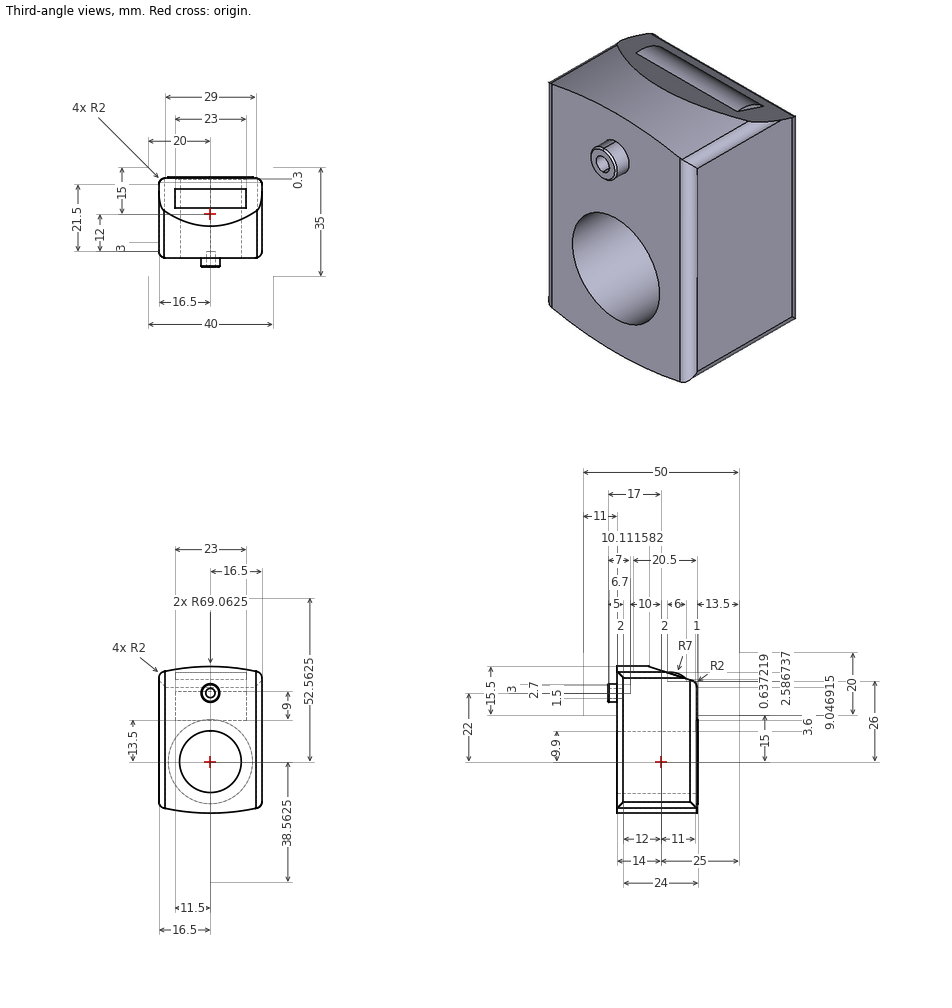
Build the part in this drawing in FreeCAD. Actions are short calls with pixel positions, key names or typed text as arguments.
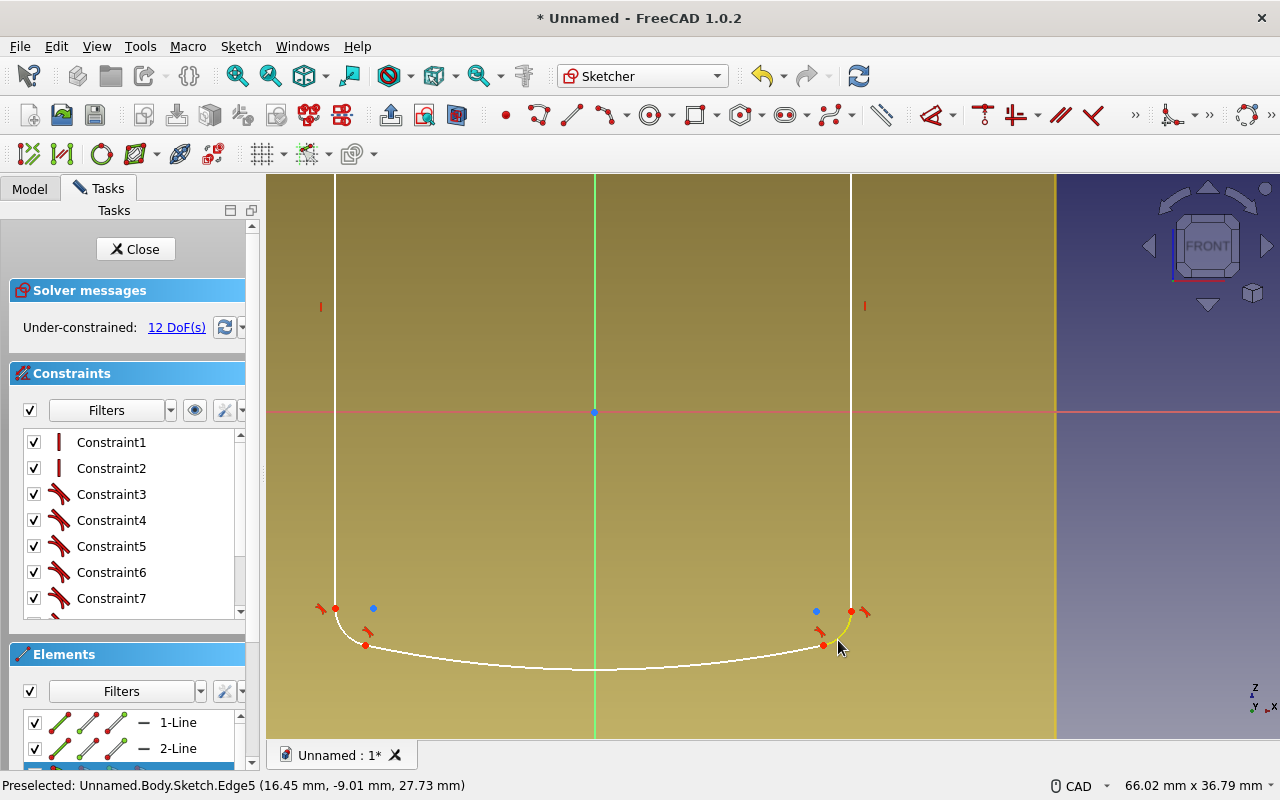
click(837, 640)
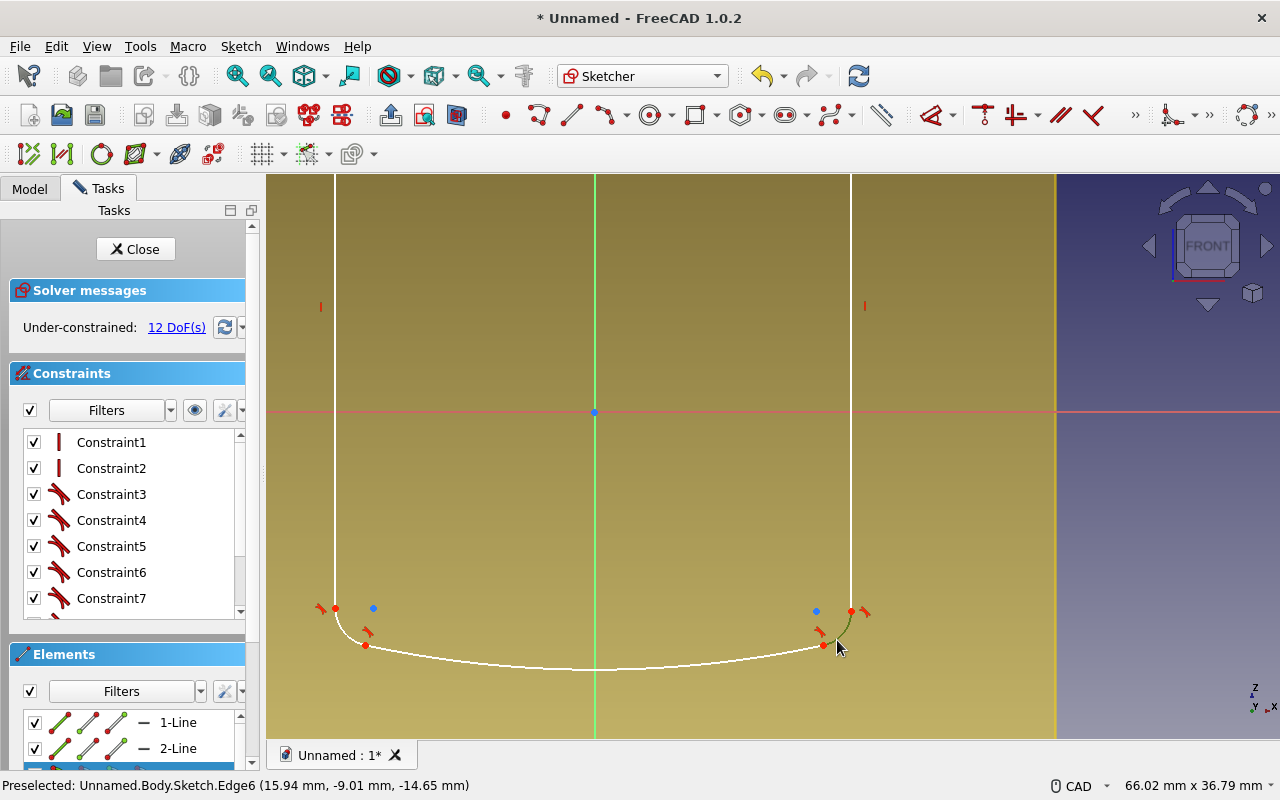
click(339, 623)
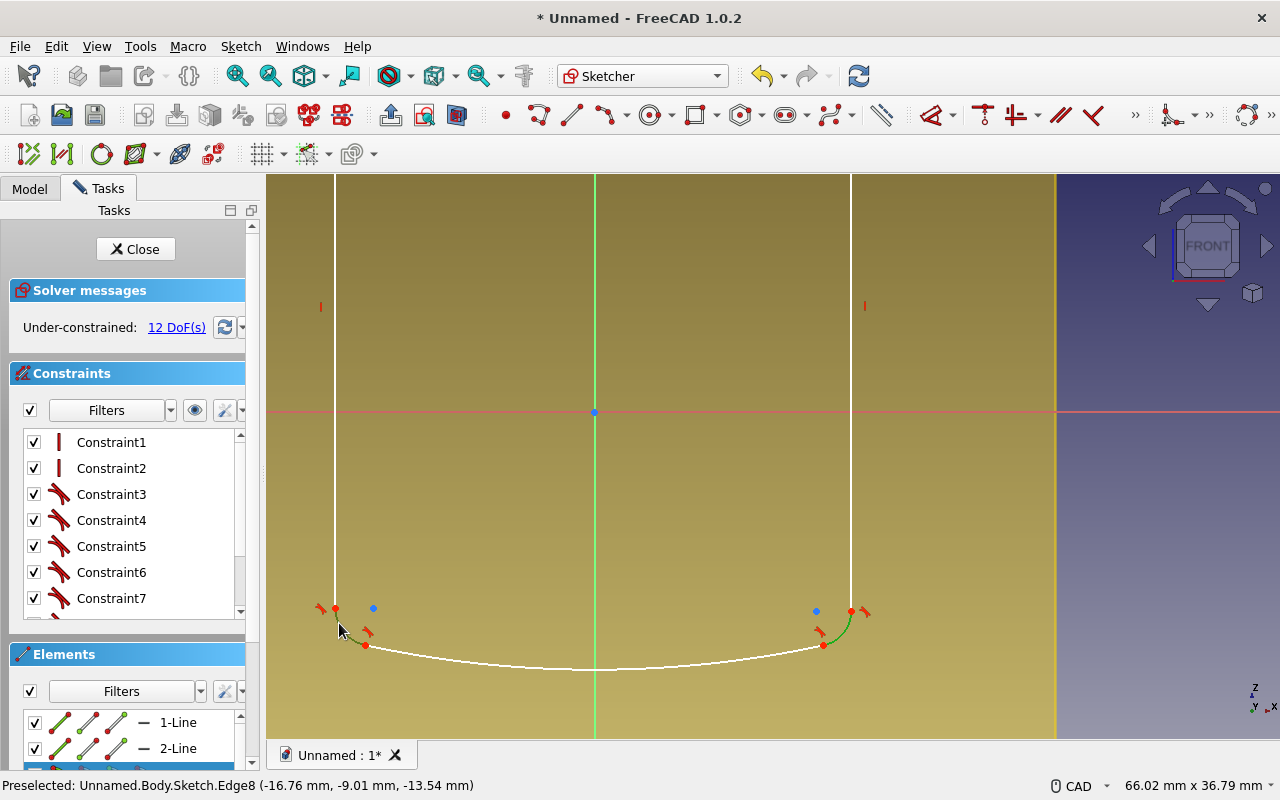
key(e)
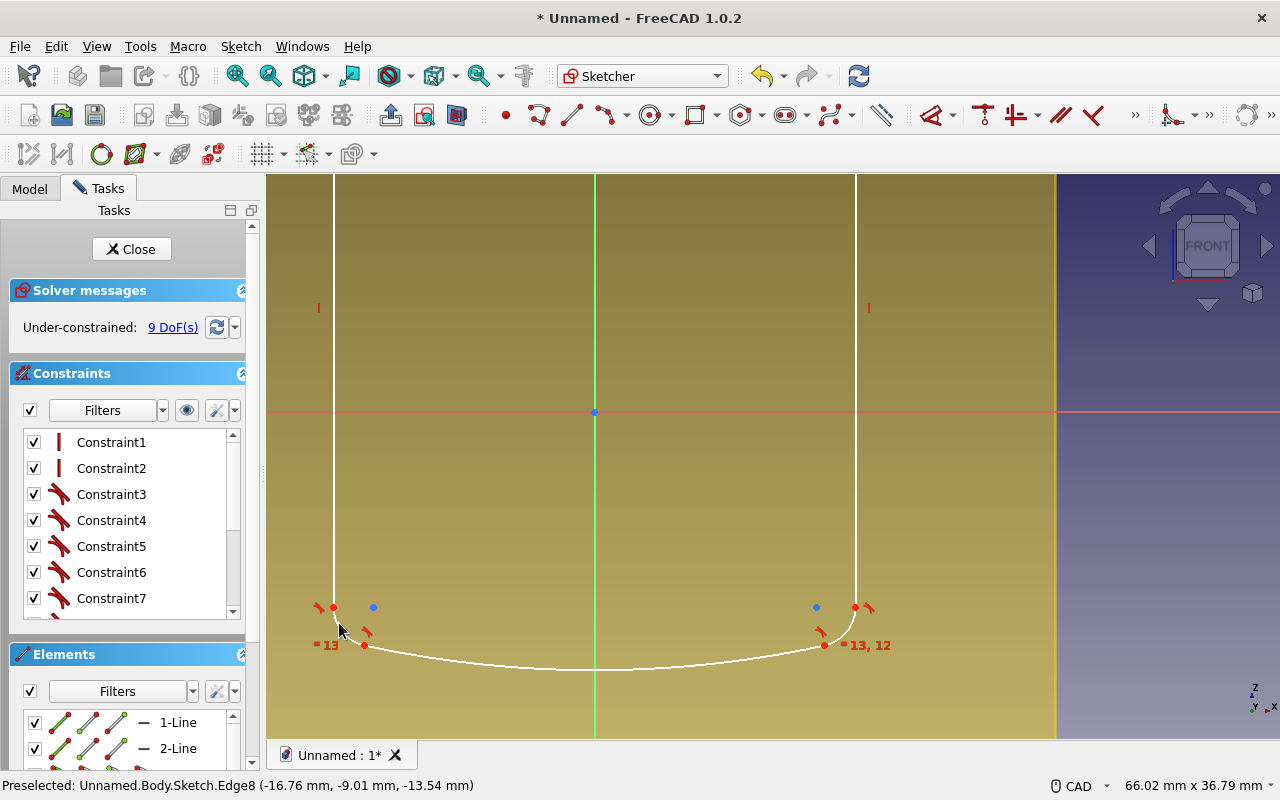
scroll(838, 641, down, 3)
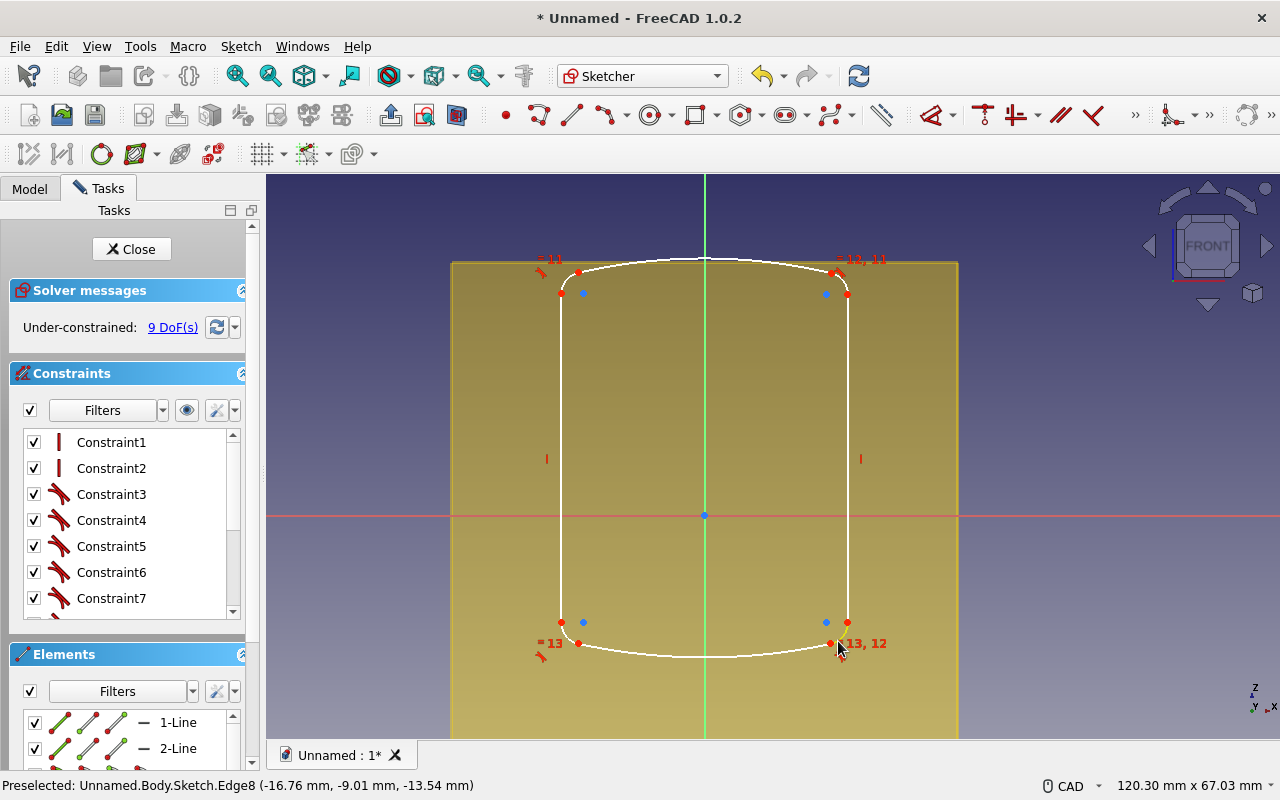
click(756, 261)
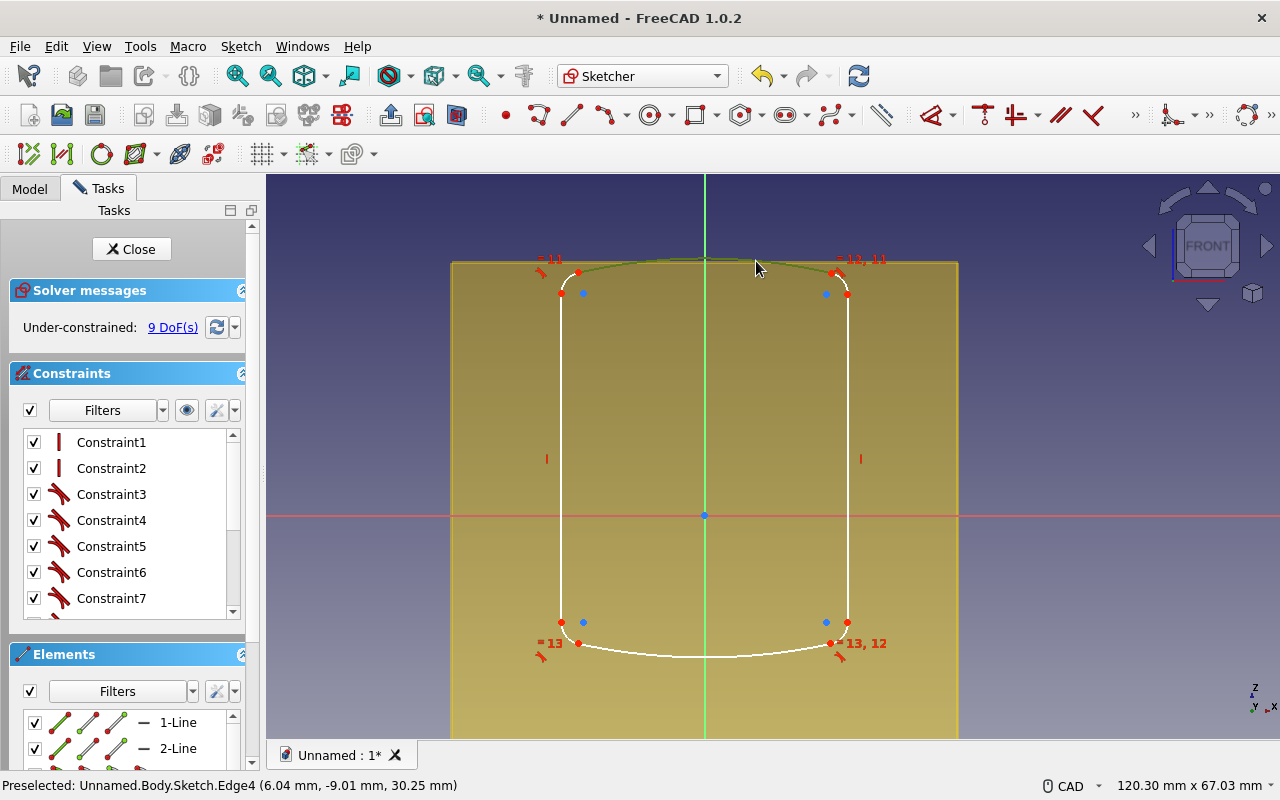
click(654, 655)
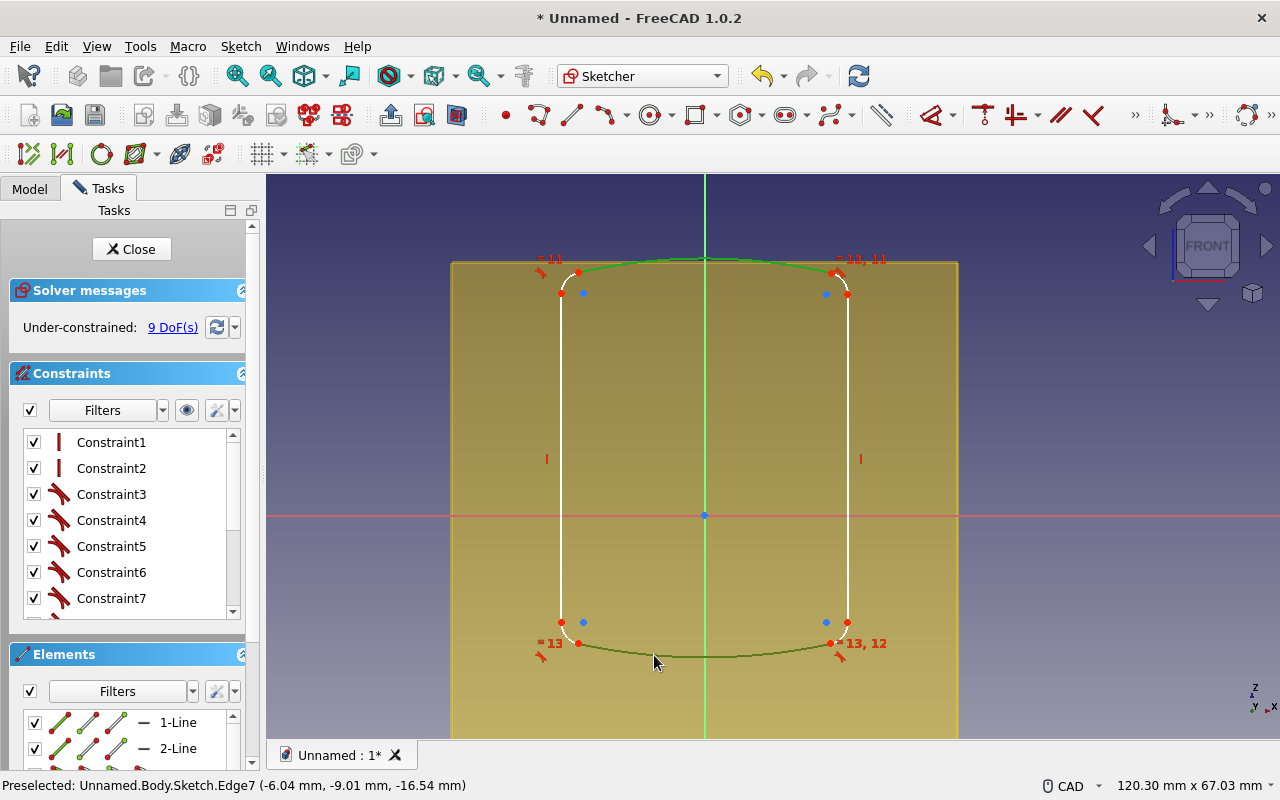
key(e)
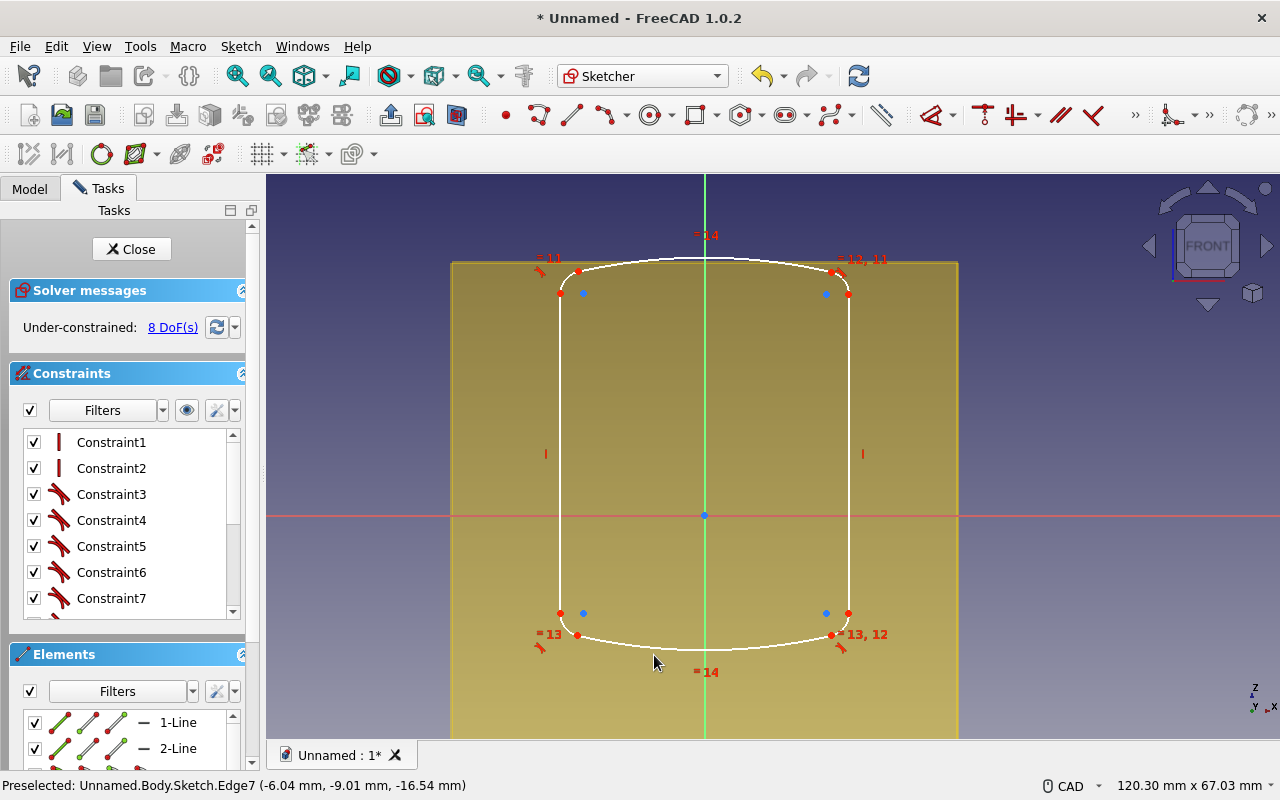
scroll(704, 283, down, 2)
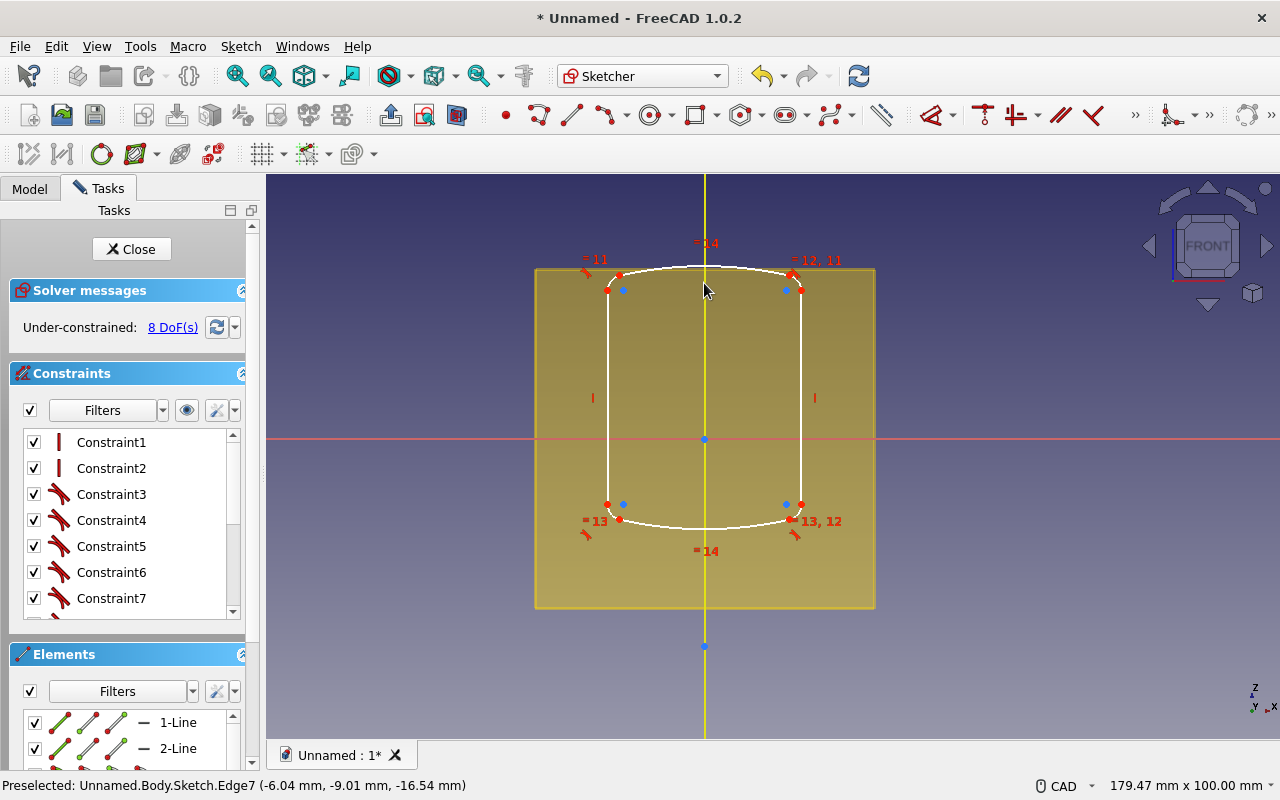
click(704, 646)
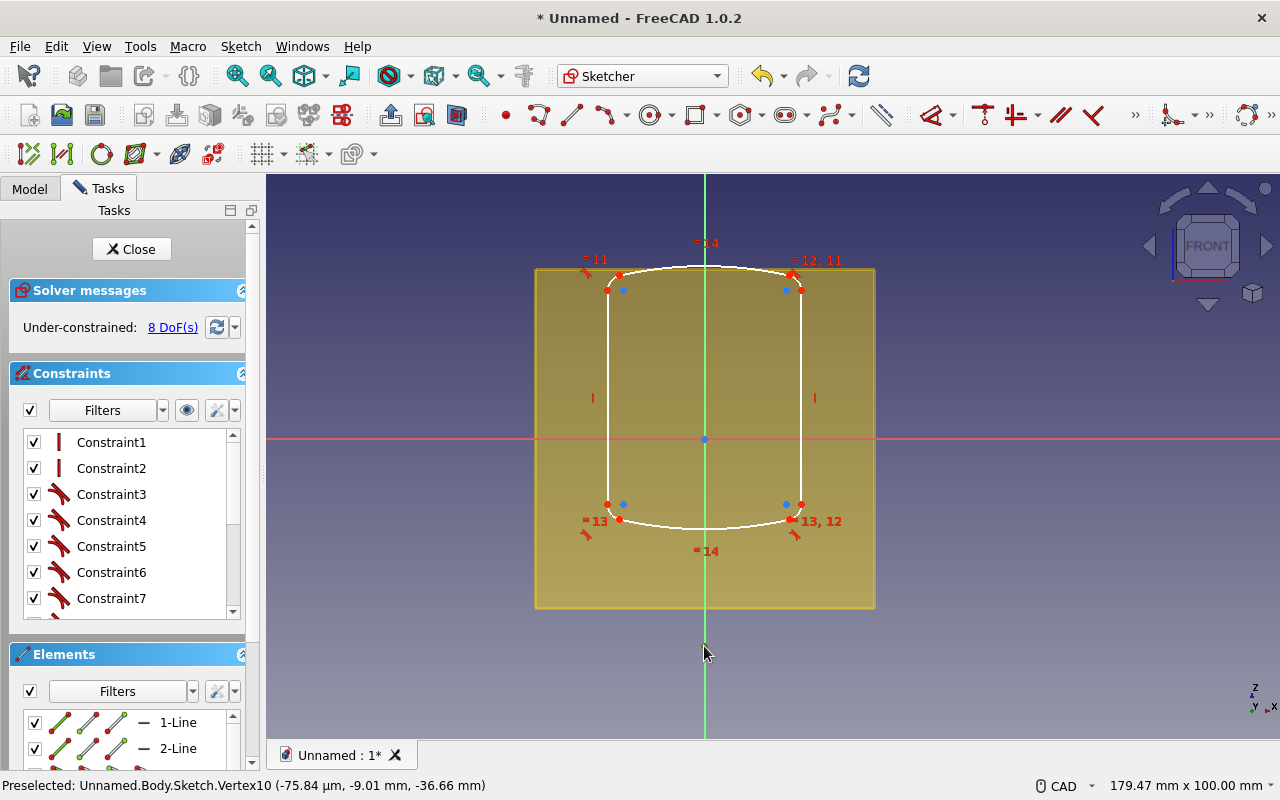
click(705, 675)